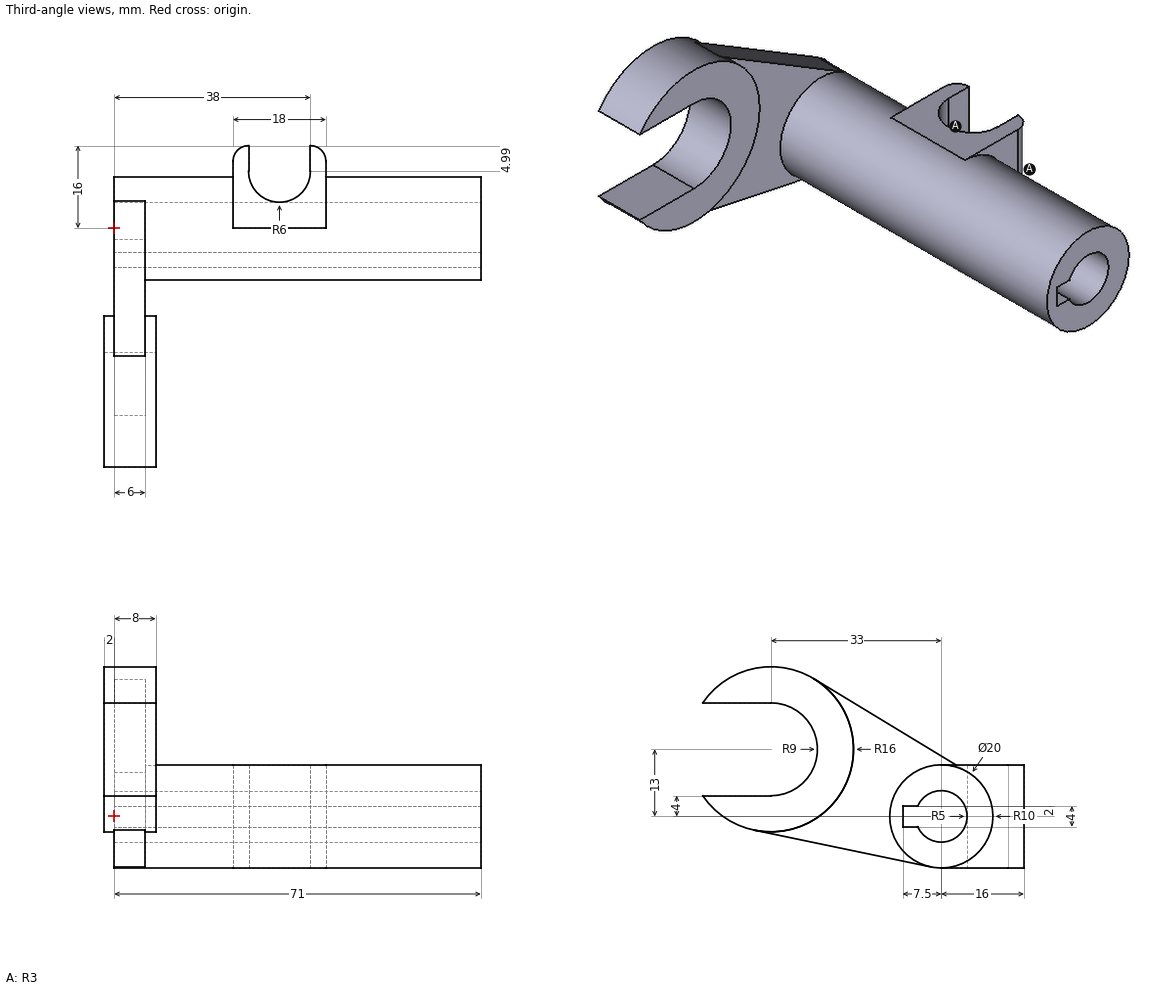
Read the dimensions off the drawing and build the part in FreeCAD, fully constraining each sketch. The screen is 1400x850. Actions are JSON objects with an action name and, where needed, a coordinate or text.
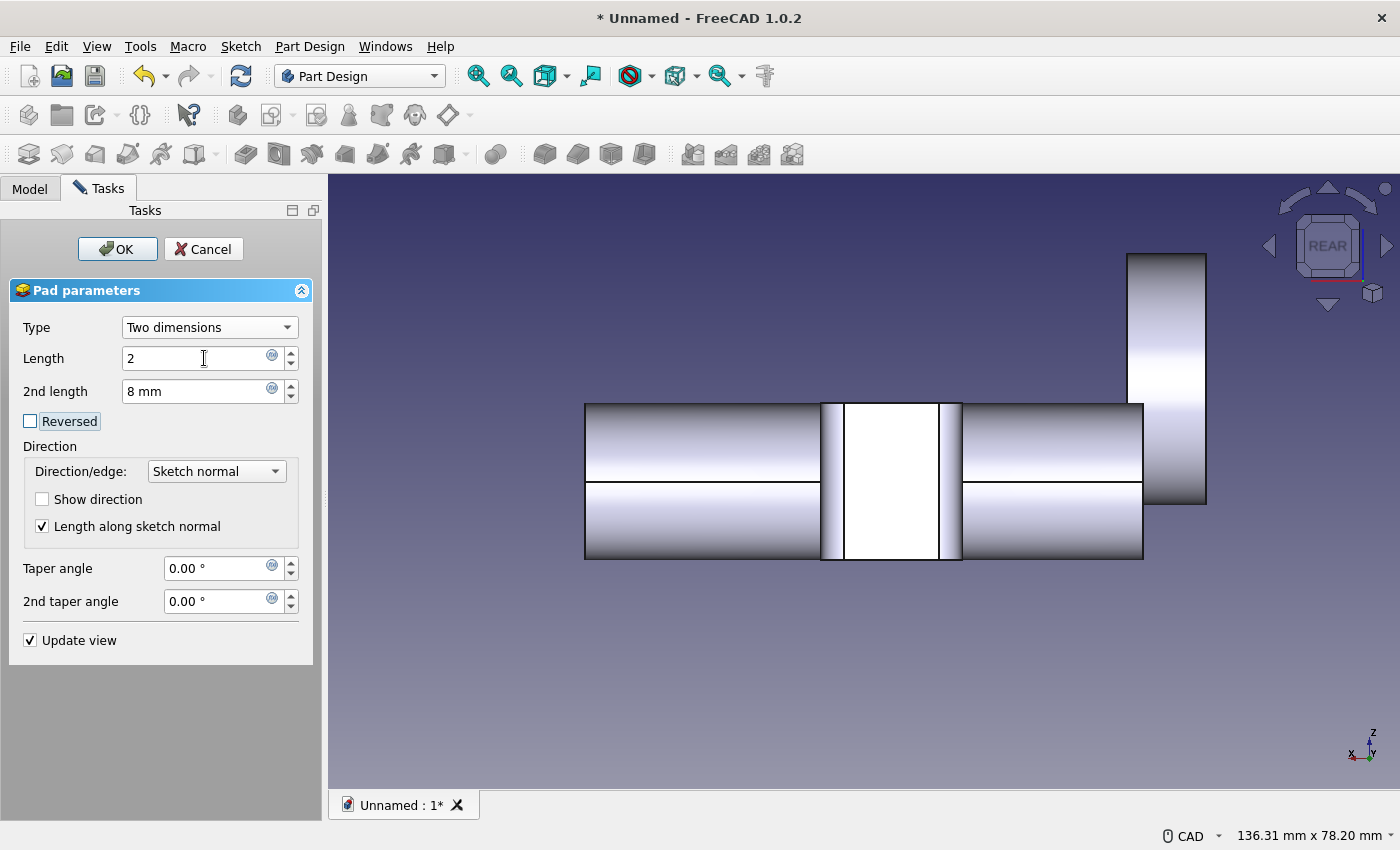
{"action": "left_click", "coordinate": [31, 421]}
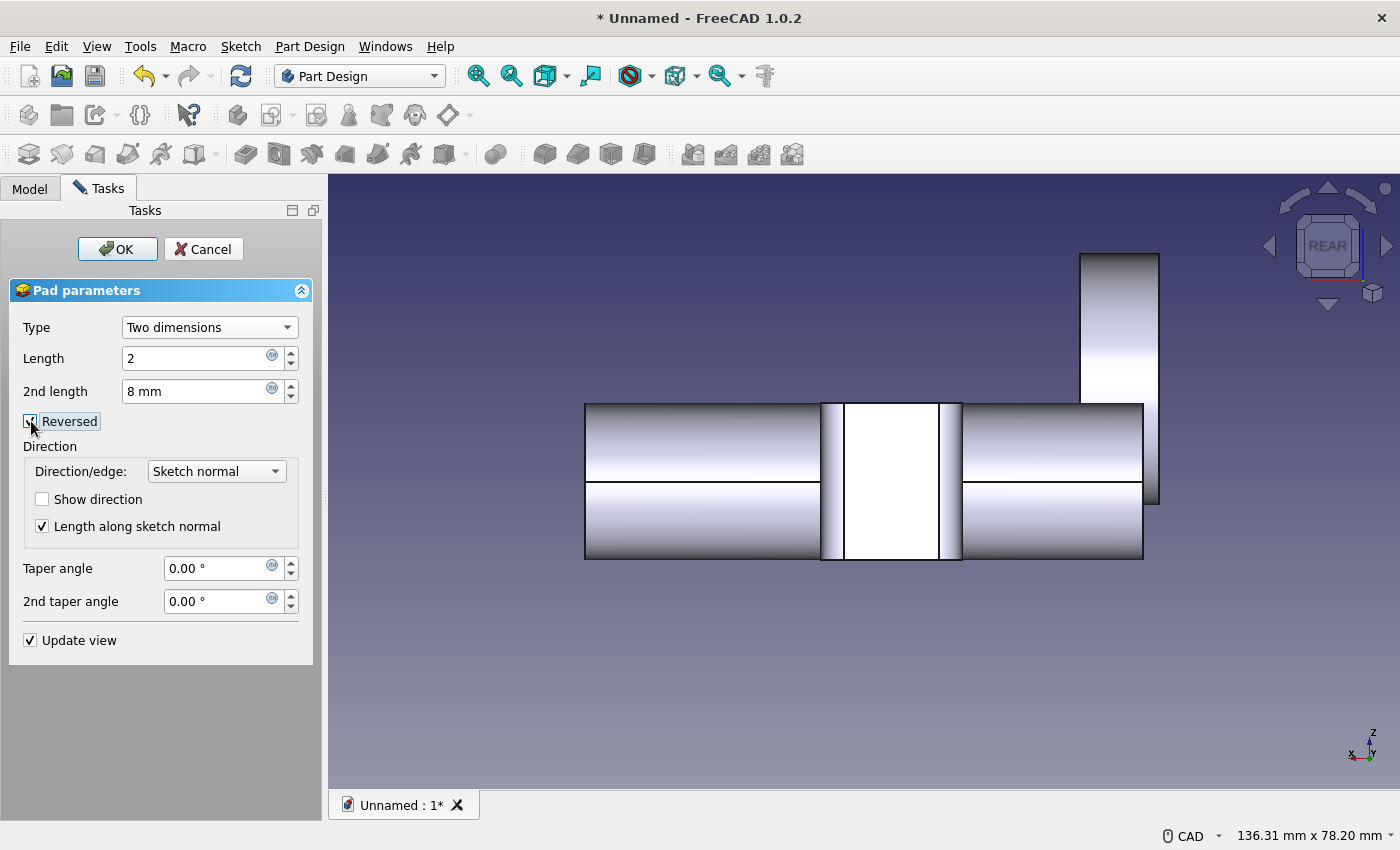
{"action": "left_click", "coordinate": [118, 249]}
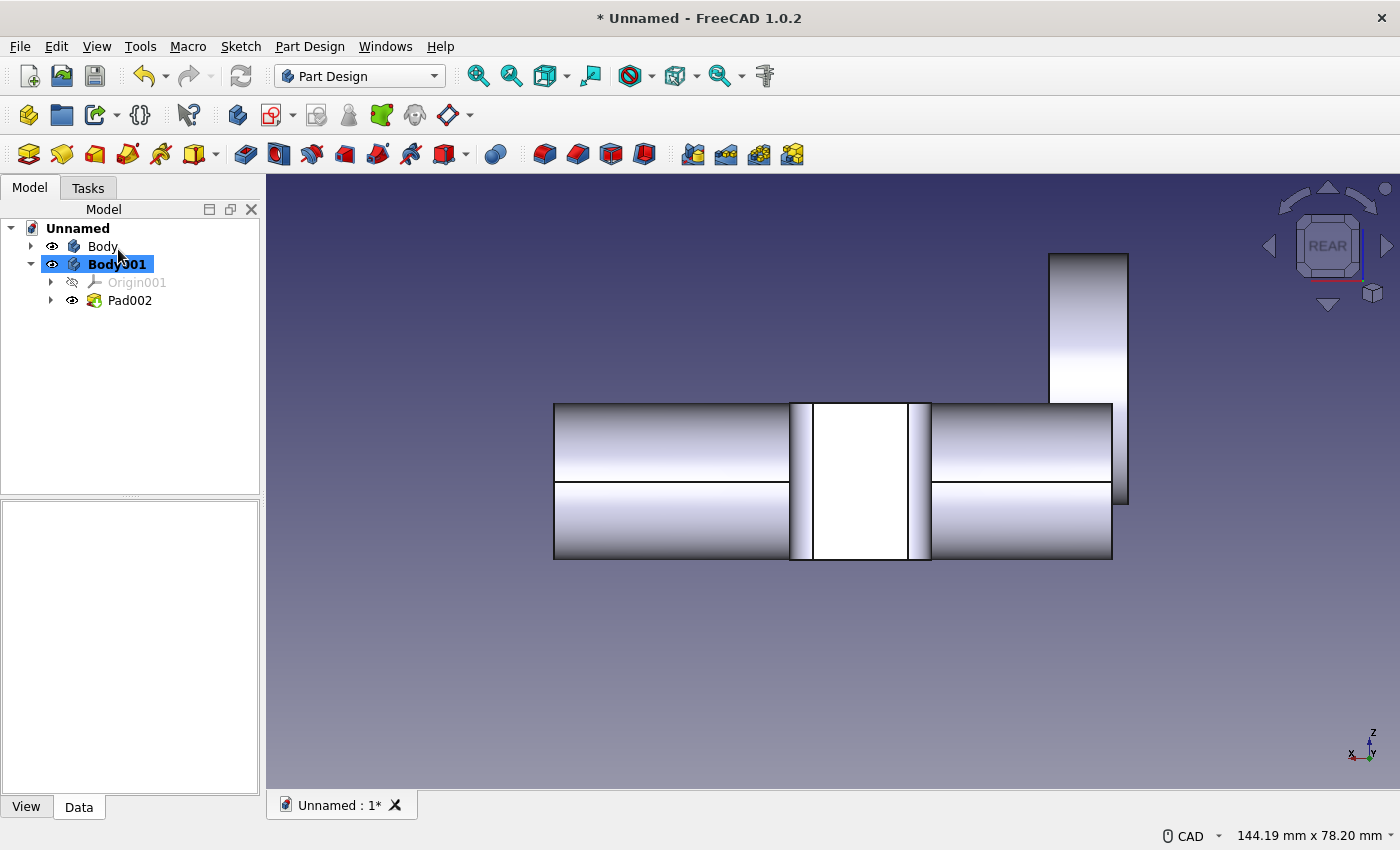
{"action": "key", "text": "v f"}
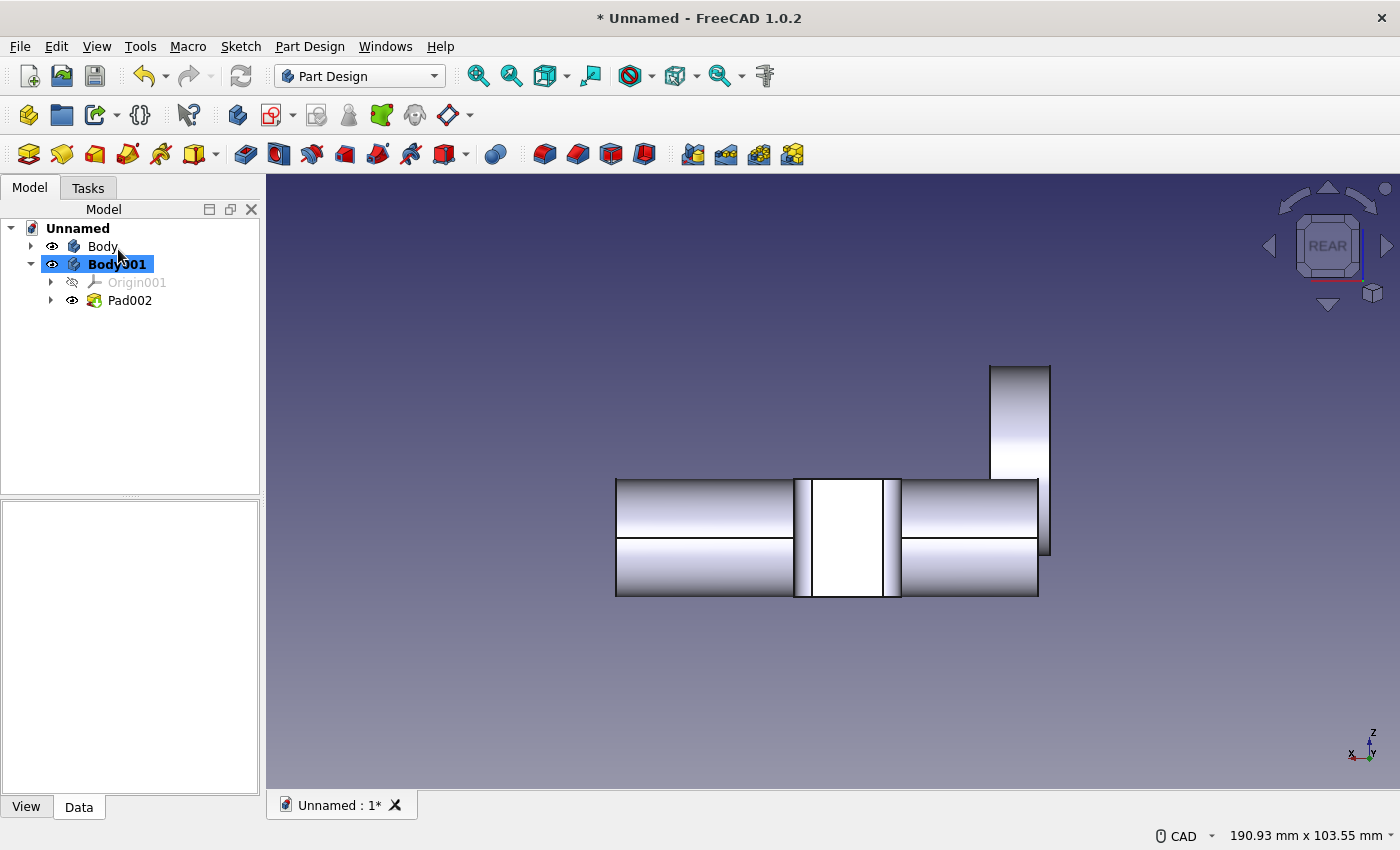
{"action": "double_click", "coordinate": [97, 246]}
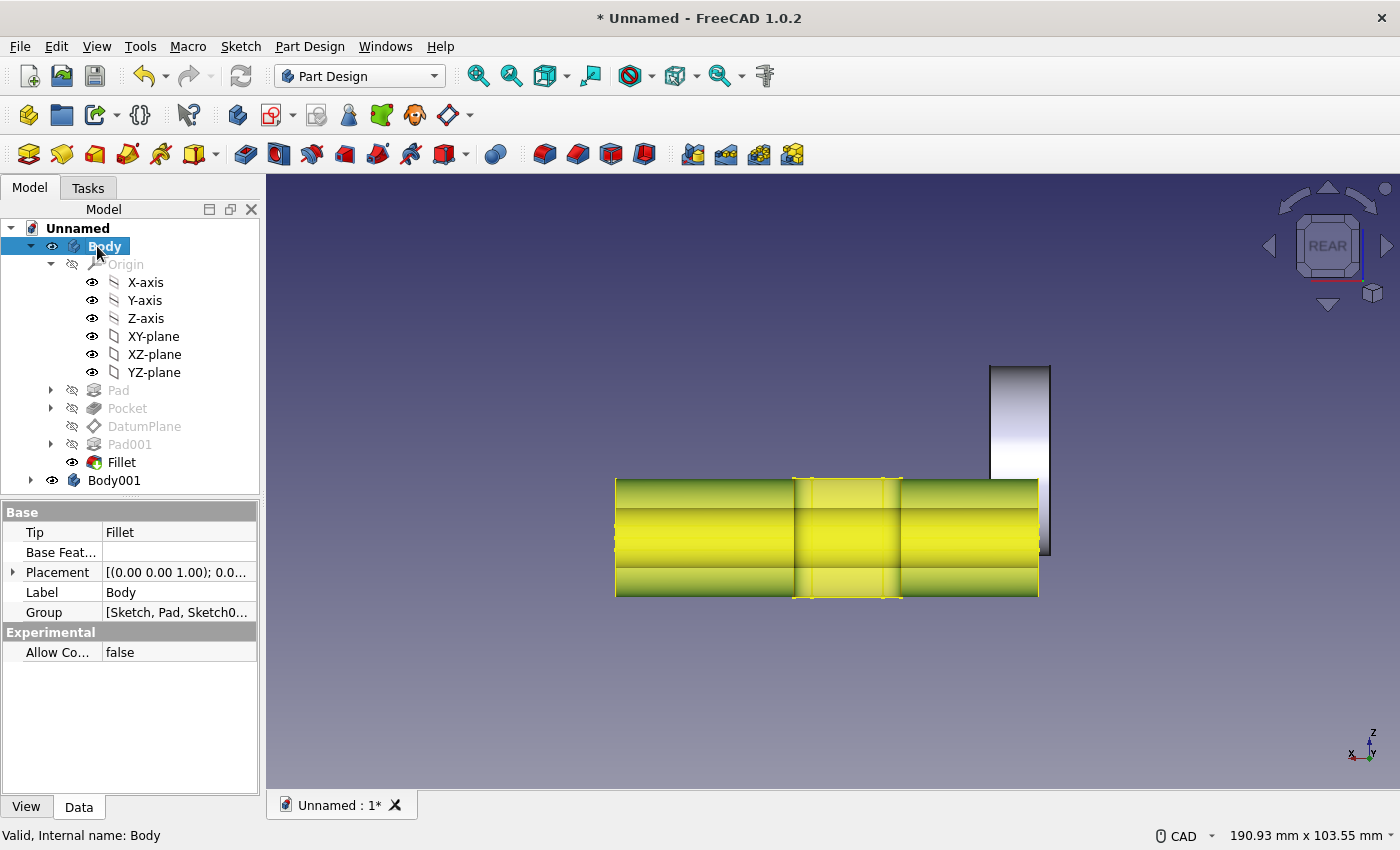
{"action": "left_click", "coordinate": [97, 246]}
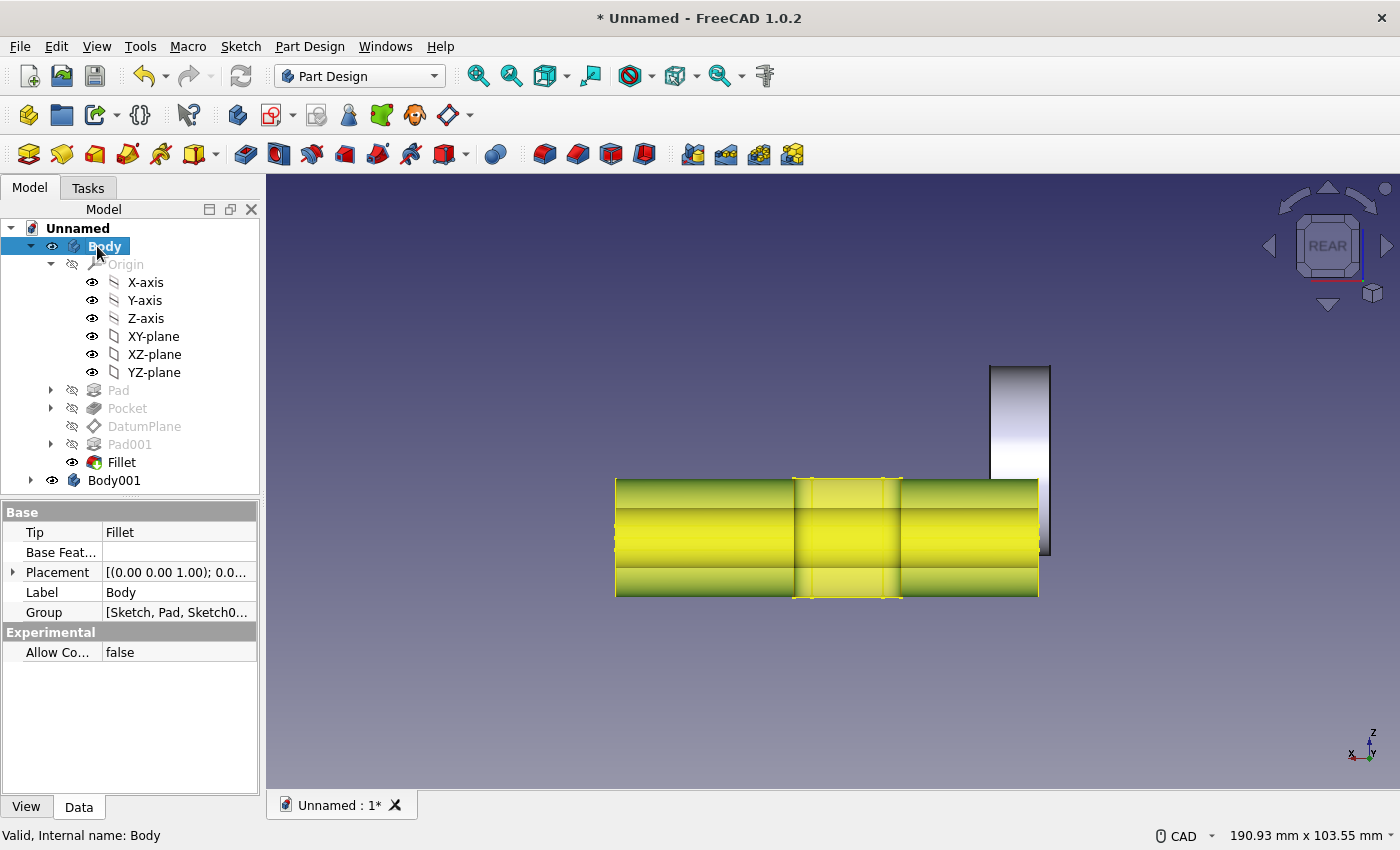
{"action": "left_click", "coordinate": [148, 652]}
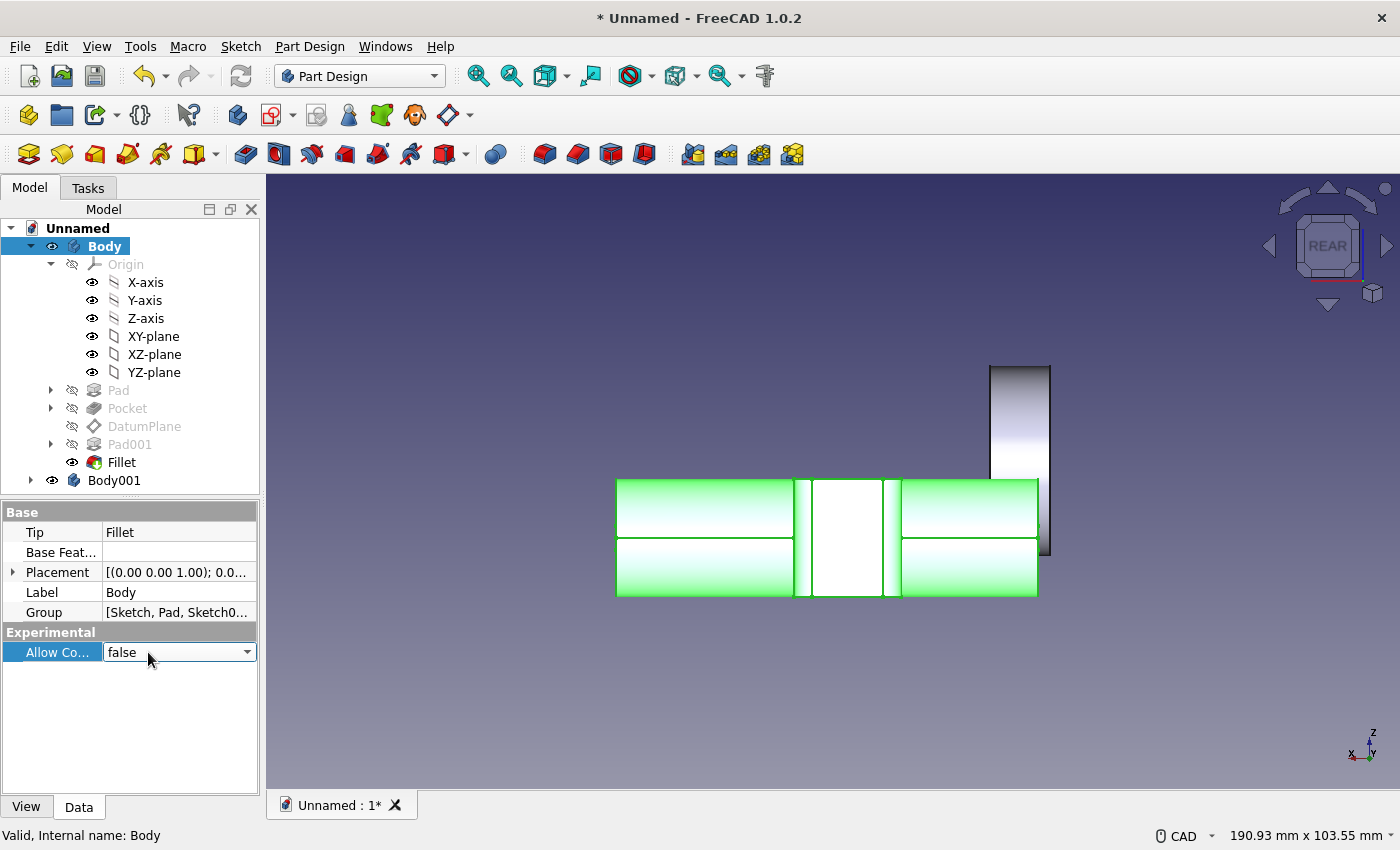
{"action": "left_click", "coordinate": [148, 652]}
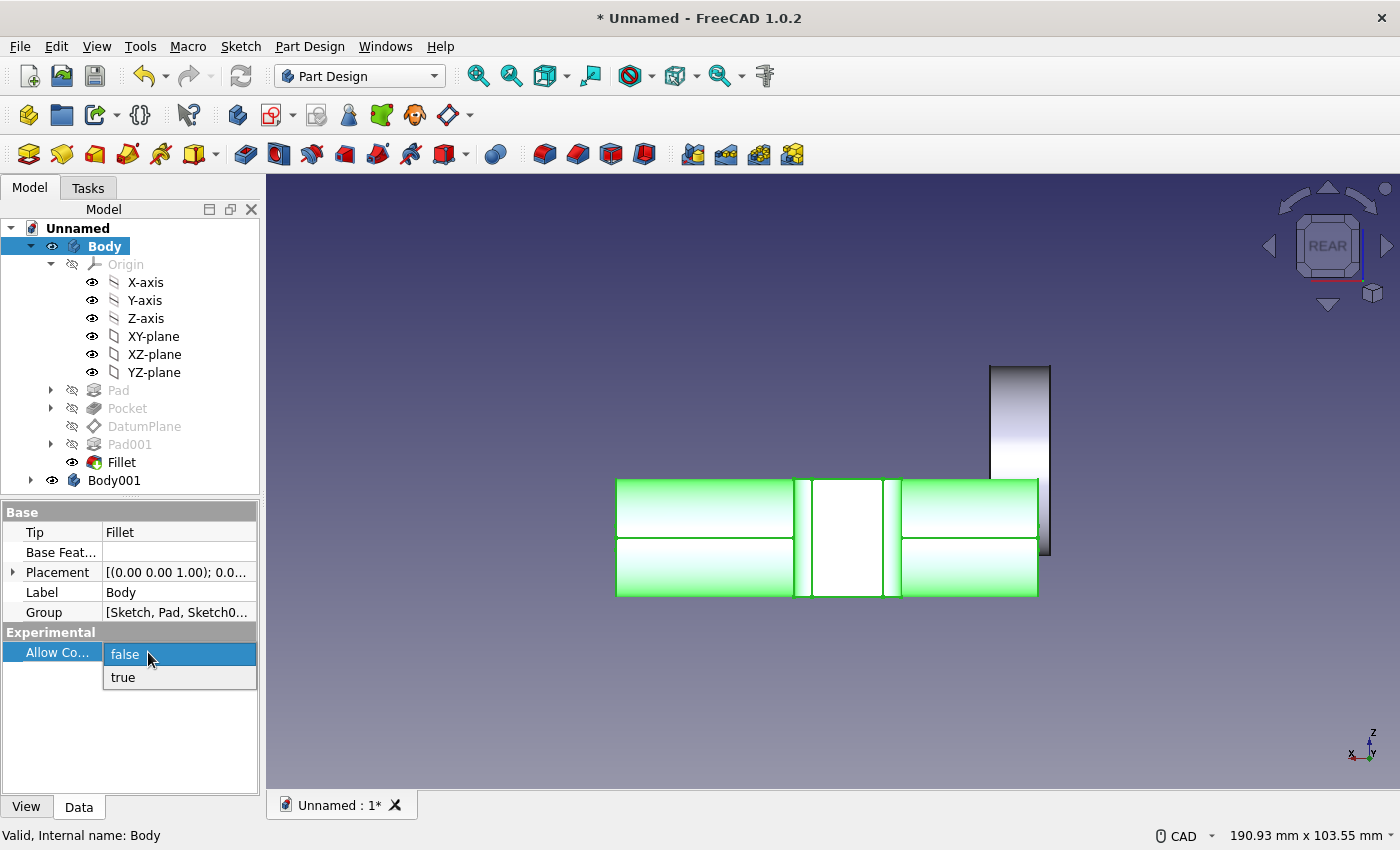
{"action": "left_click", "coordinate": [178, 678]}
{"action": "key", "text": "Return"}